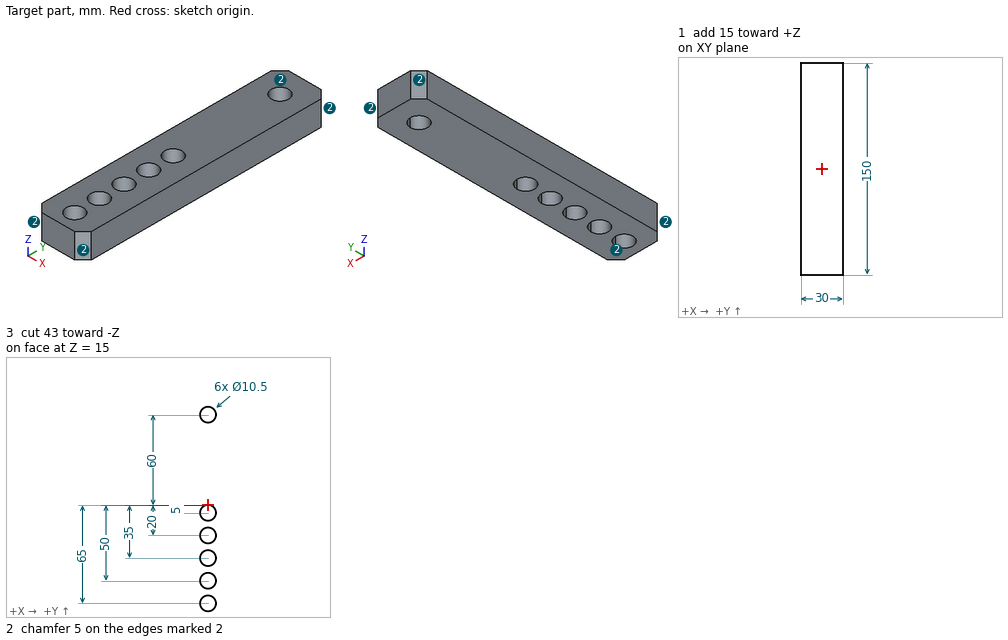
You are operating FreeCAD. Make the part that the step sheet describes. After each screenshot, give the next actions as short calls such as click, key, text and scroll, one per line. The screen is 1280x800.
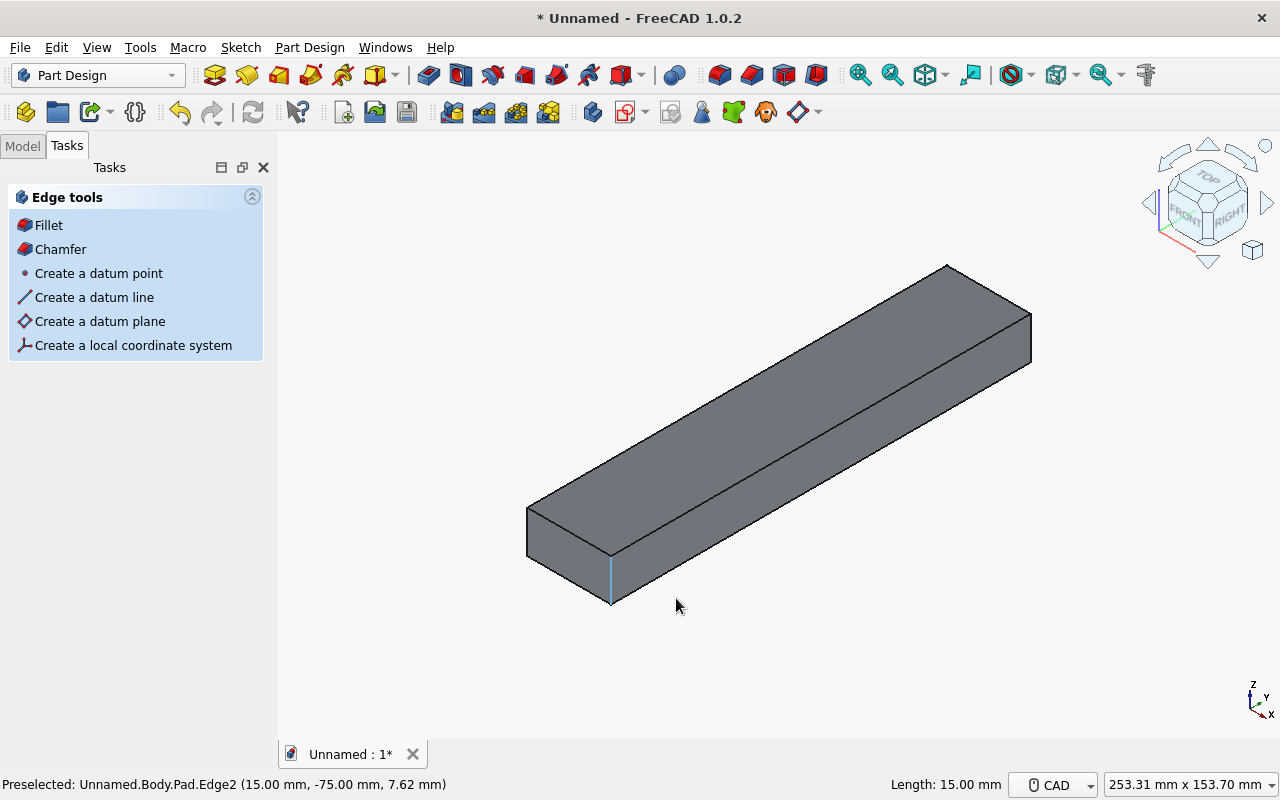
key(2)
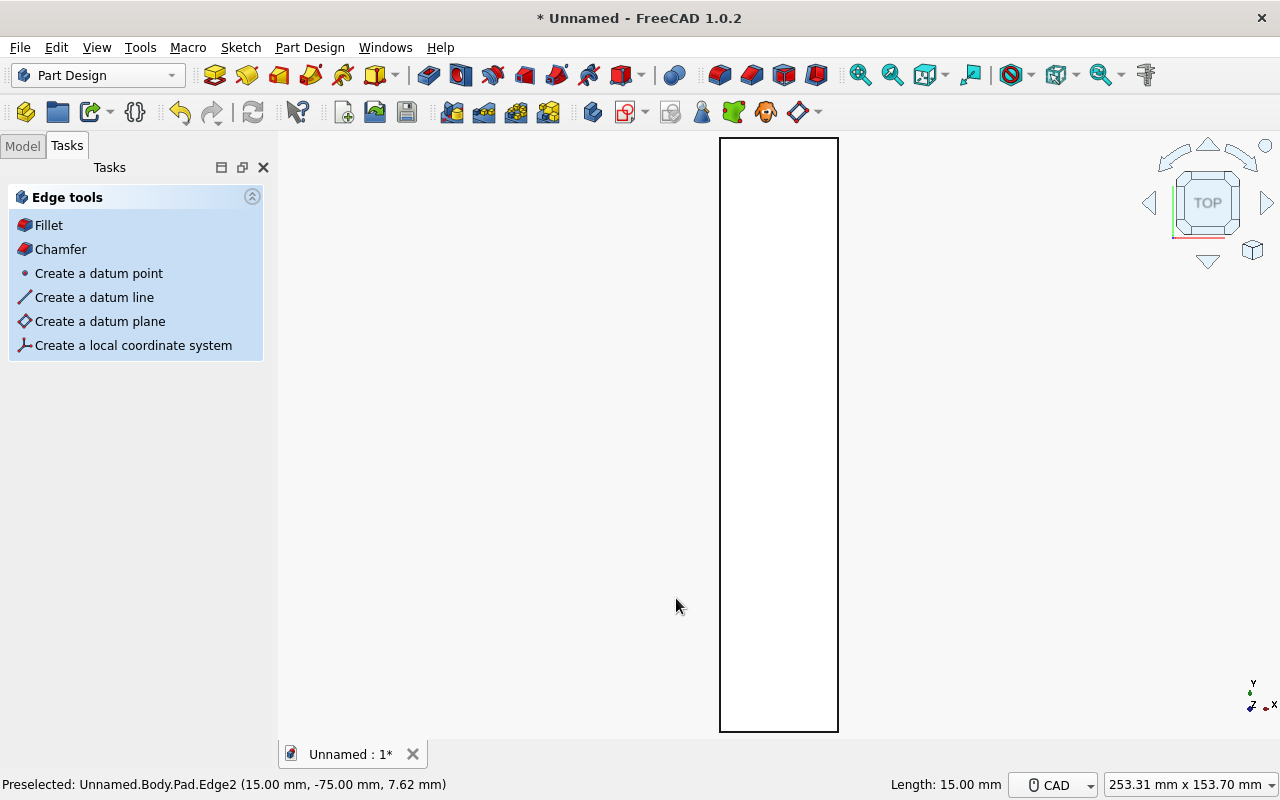
key(1)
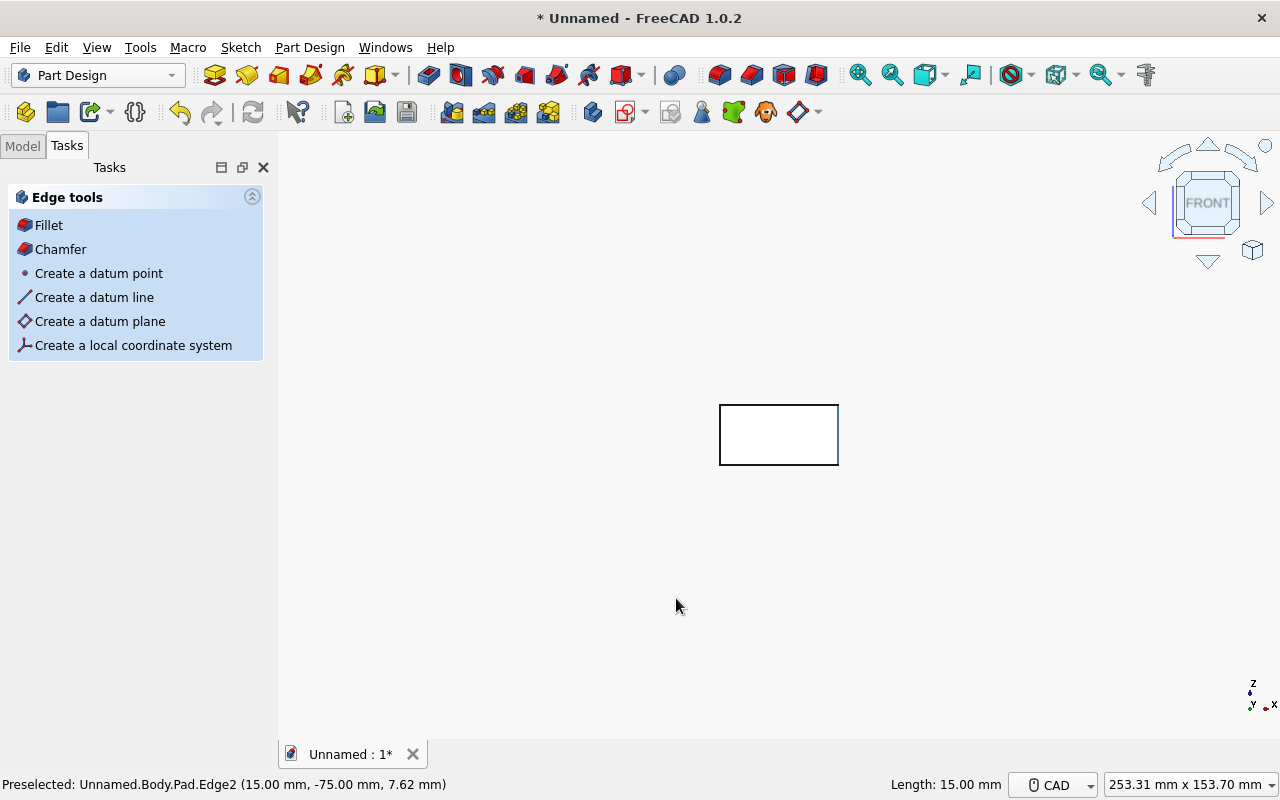
click(862, 76)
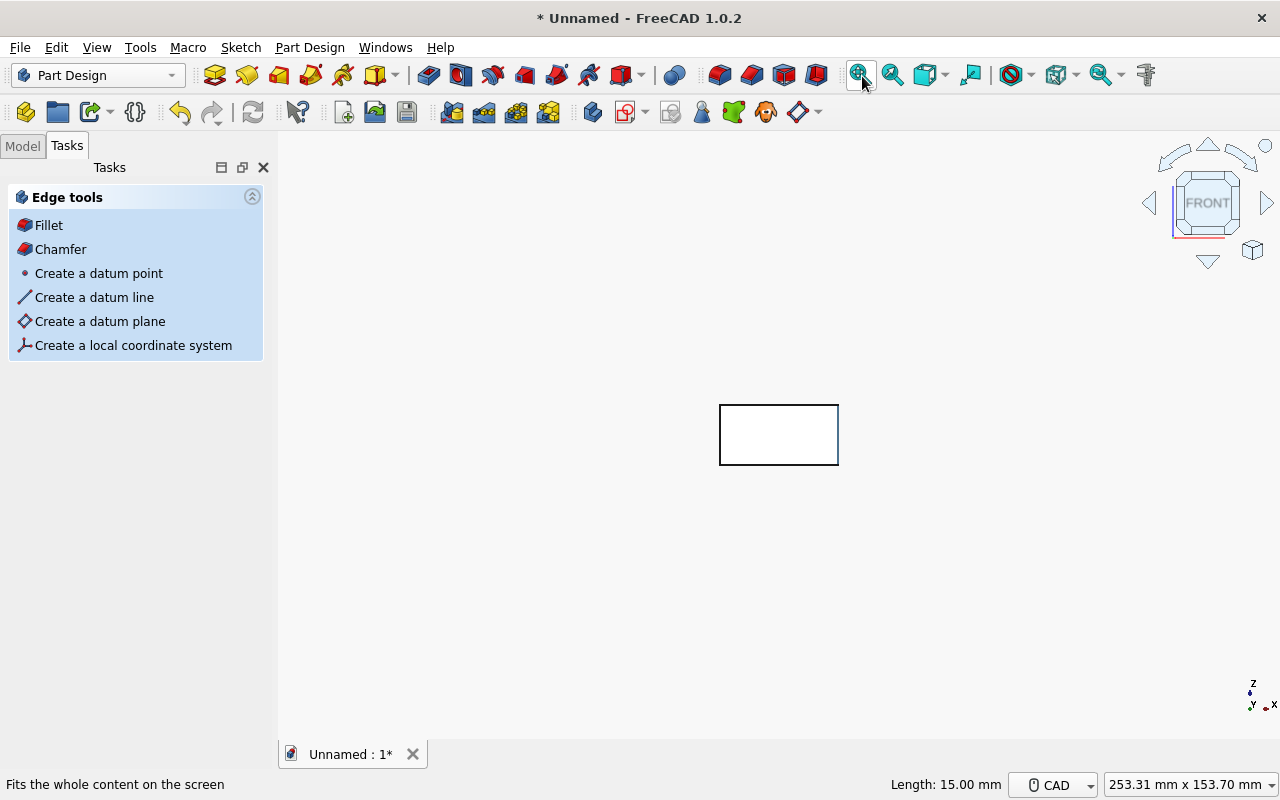
click(720, 434, ctrl)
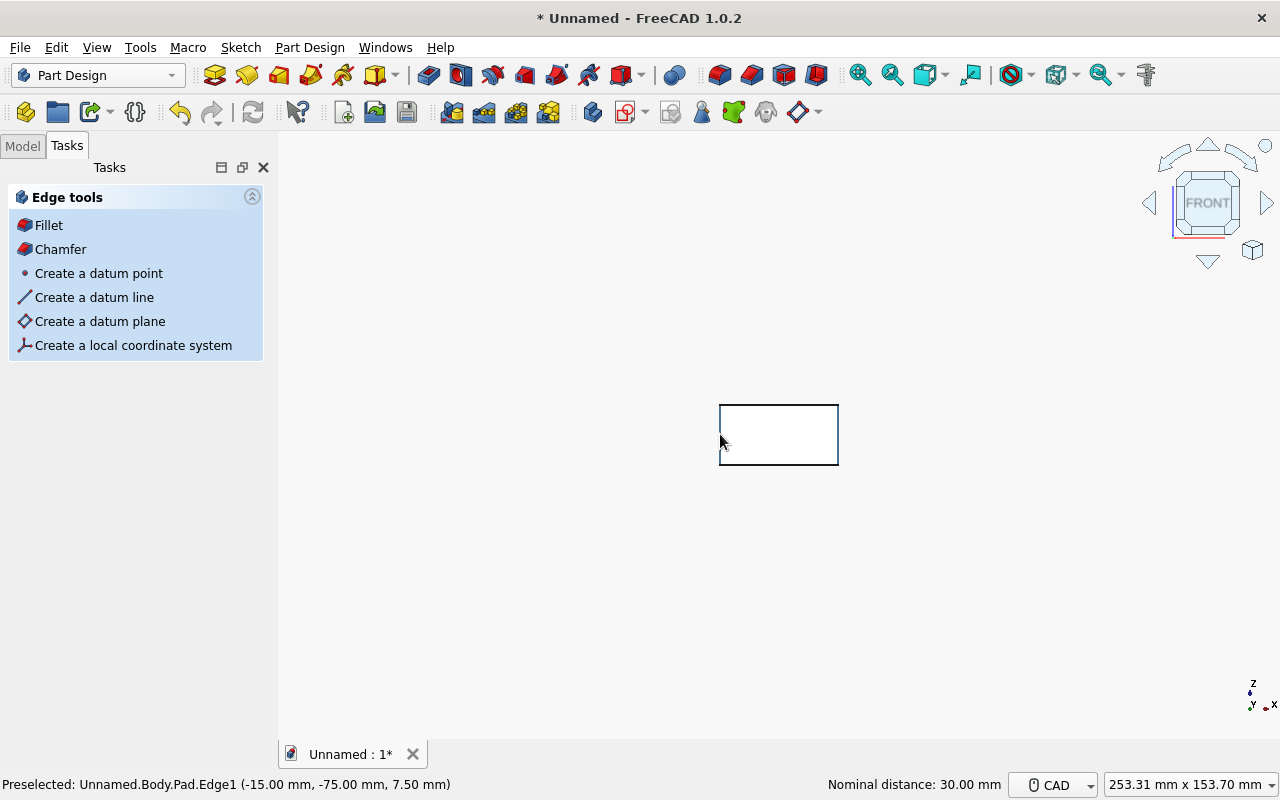
key(3)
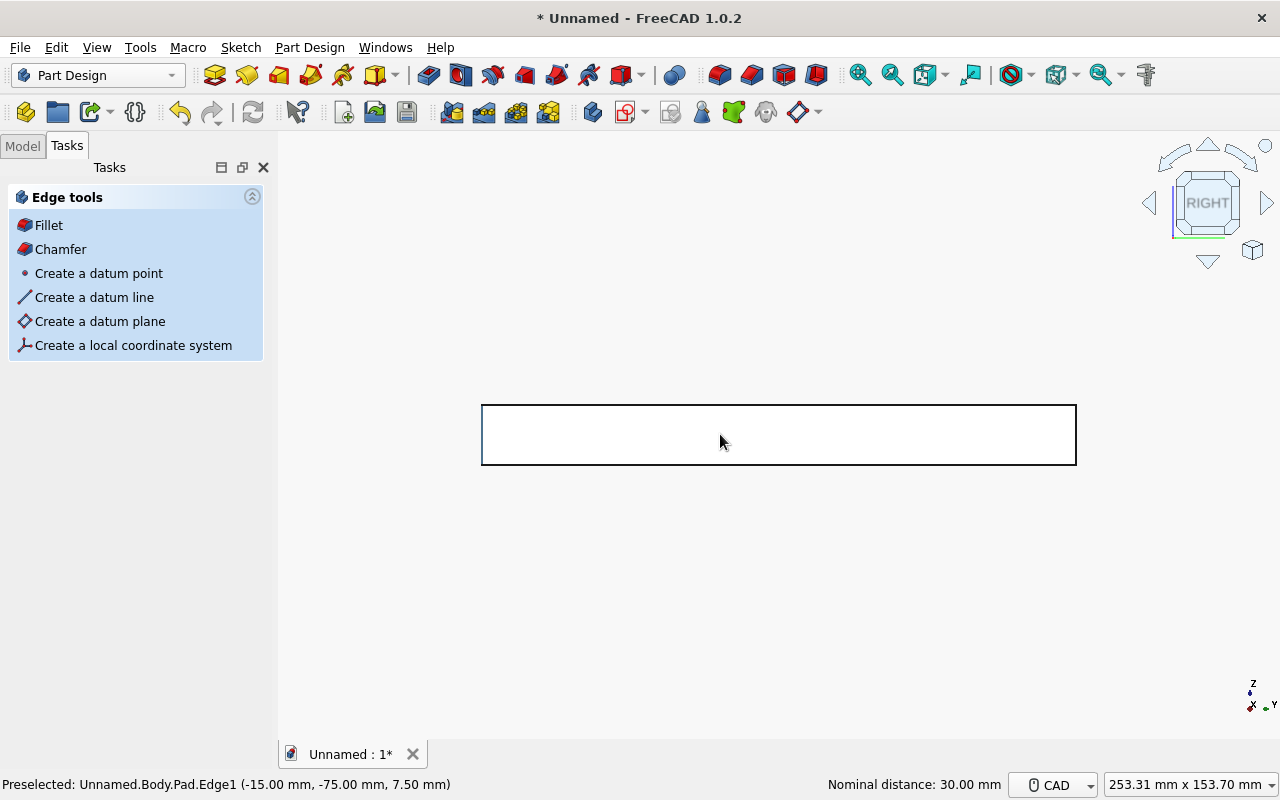
click(1076, 434, ctrl)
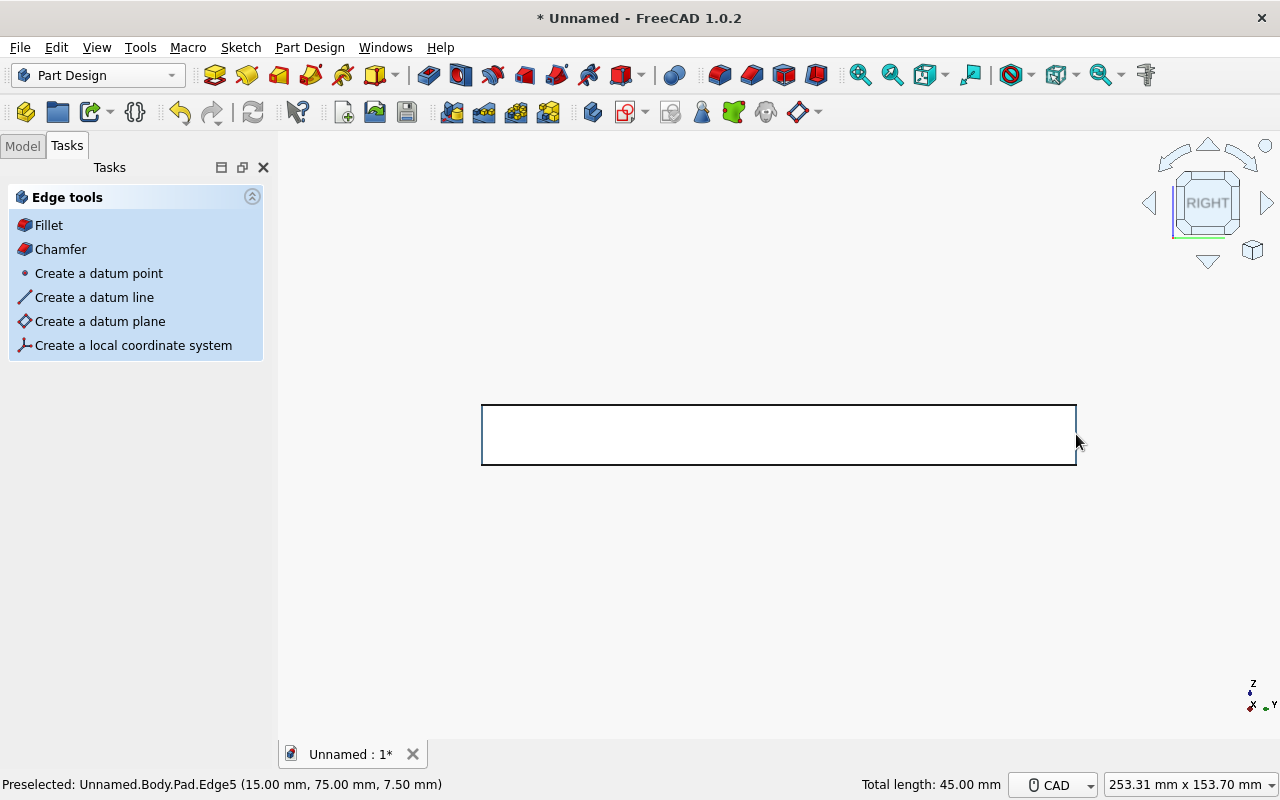
key(5)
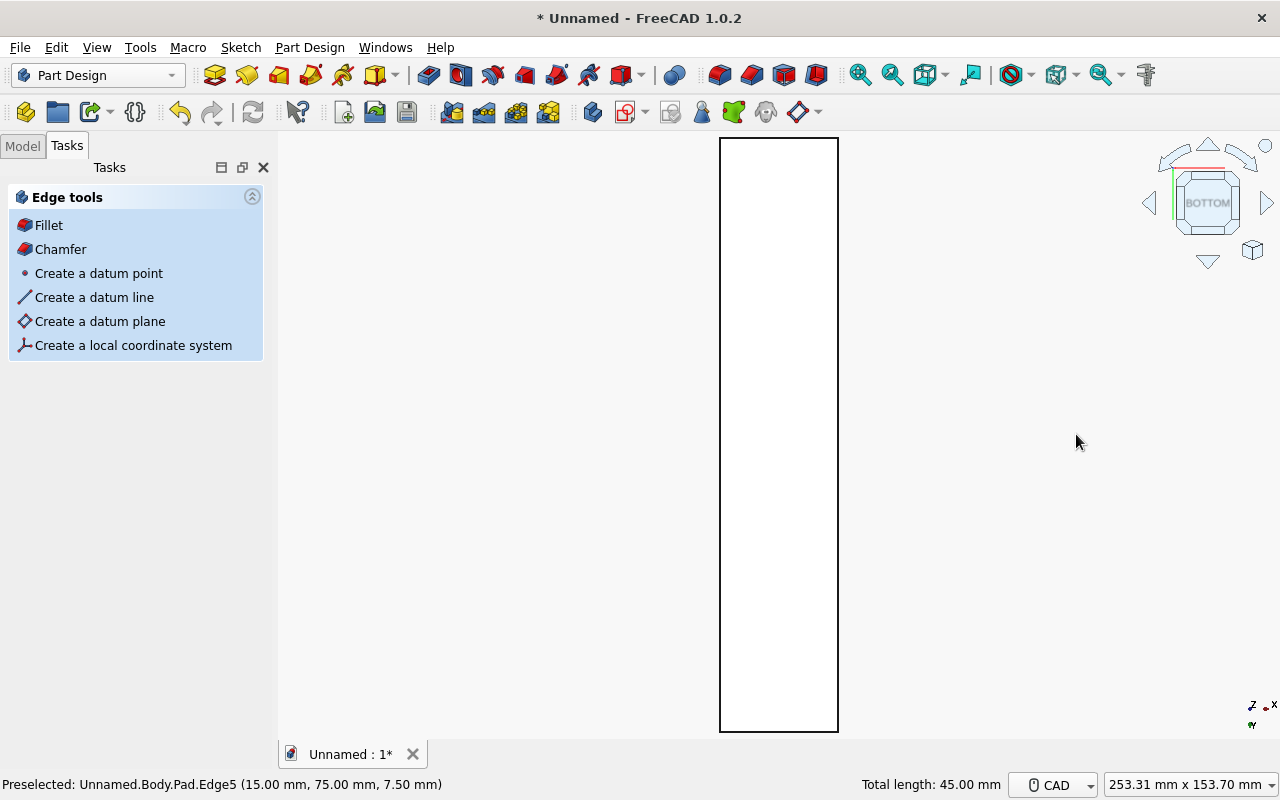
key(4)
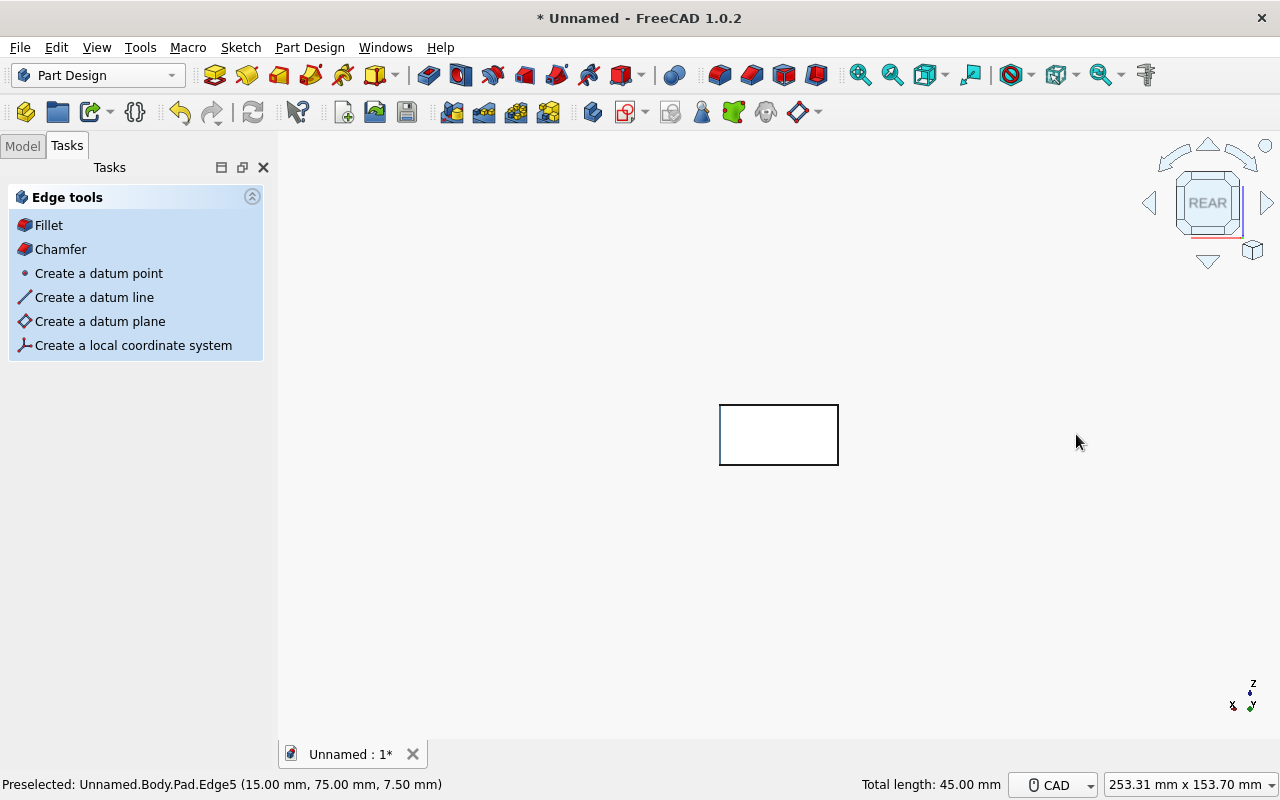
click(862, 76)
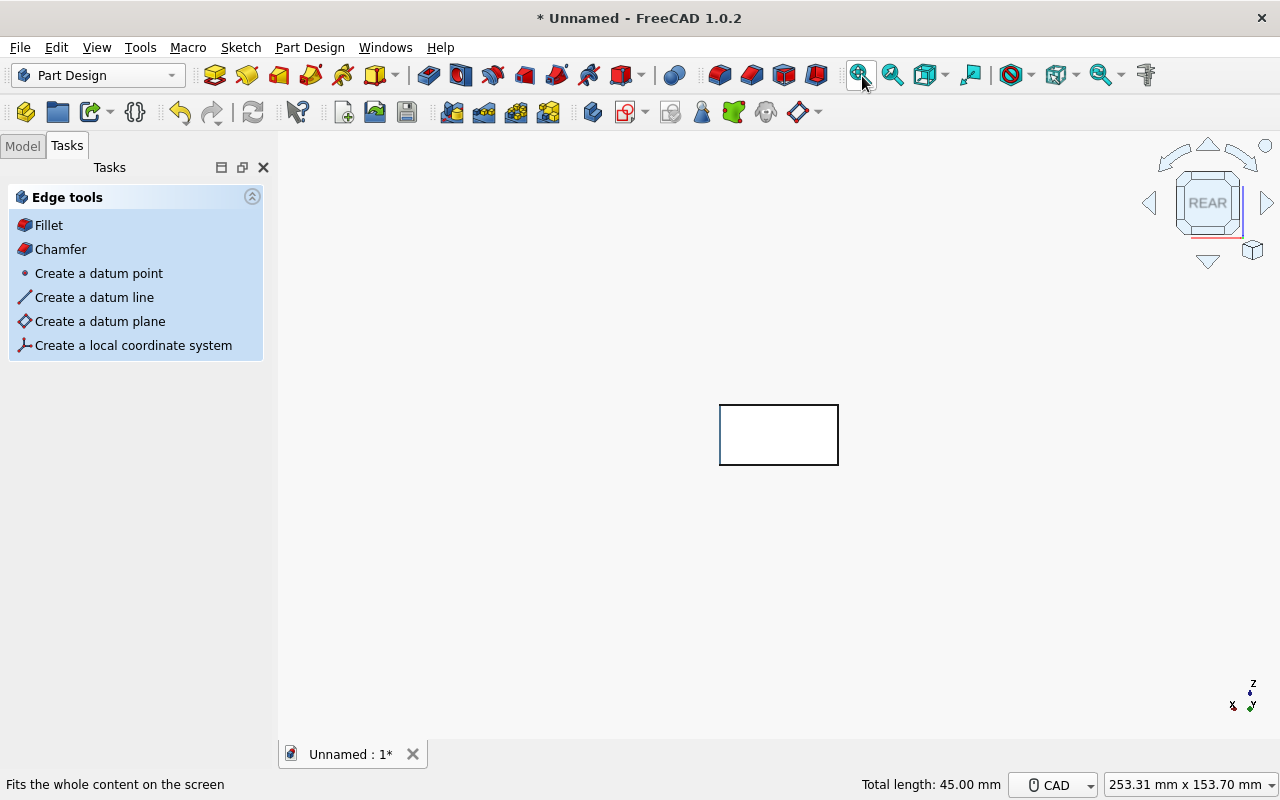
click(838, 434, ctrl)